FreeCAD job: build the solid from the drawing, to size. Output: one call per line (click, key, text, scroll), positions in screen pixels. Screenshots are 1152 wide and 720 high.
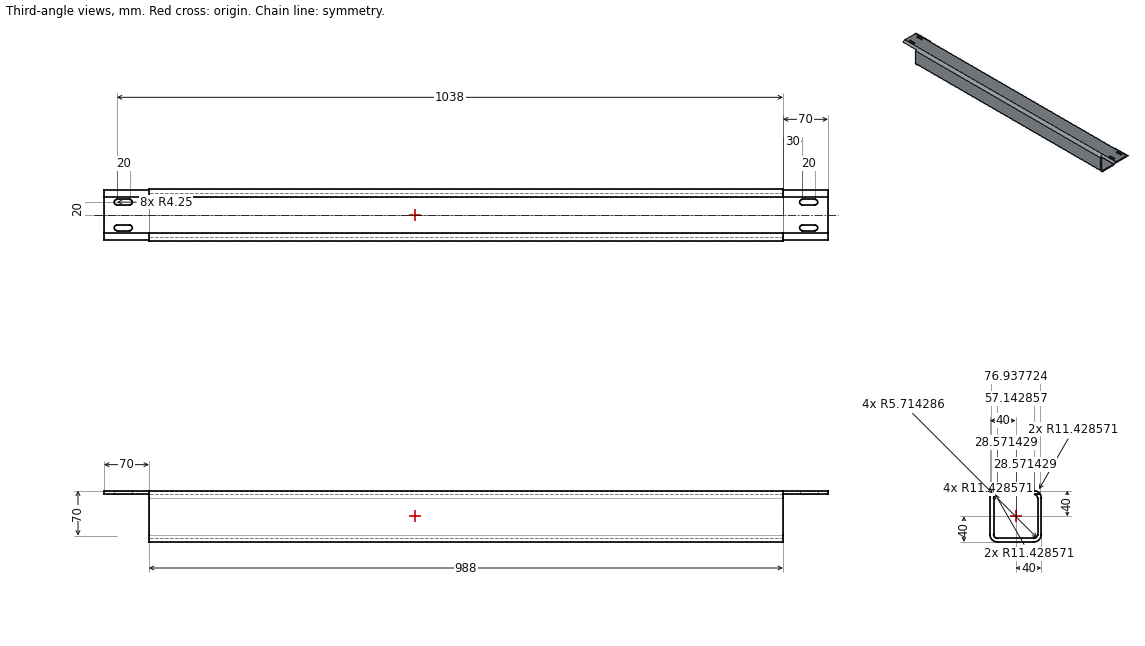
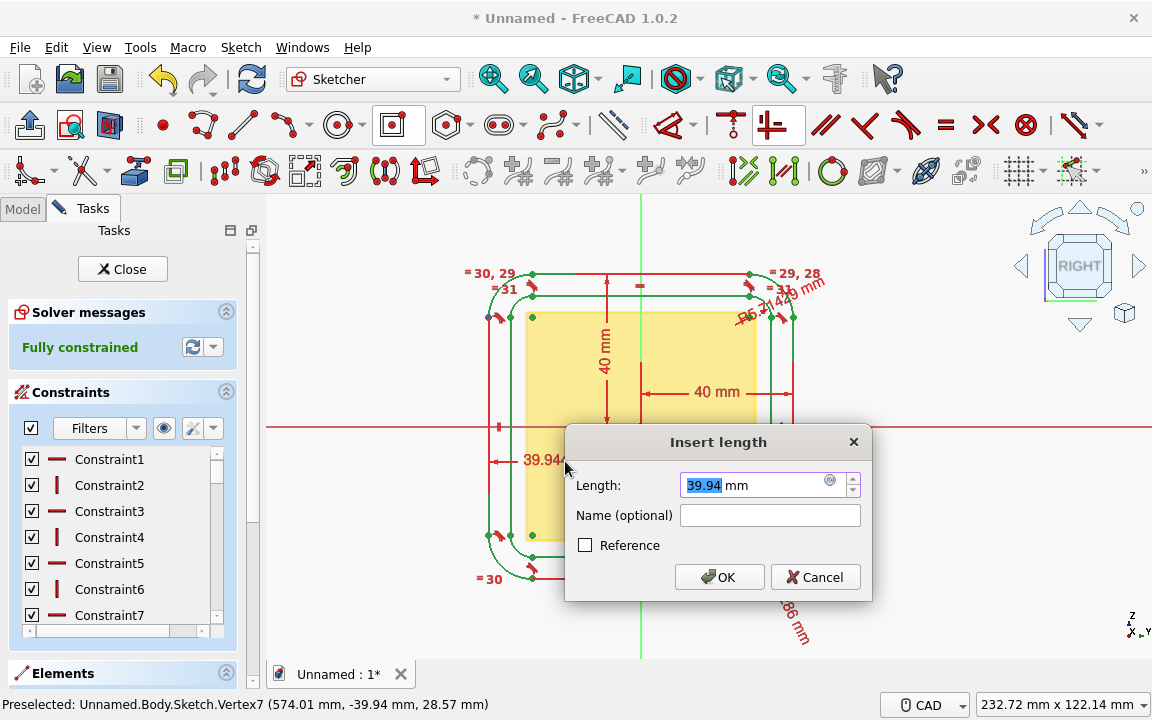
text(40)
key(Return)
key(Escape)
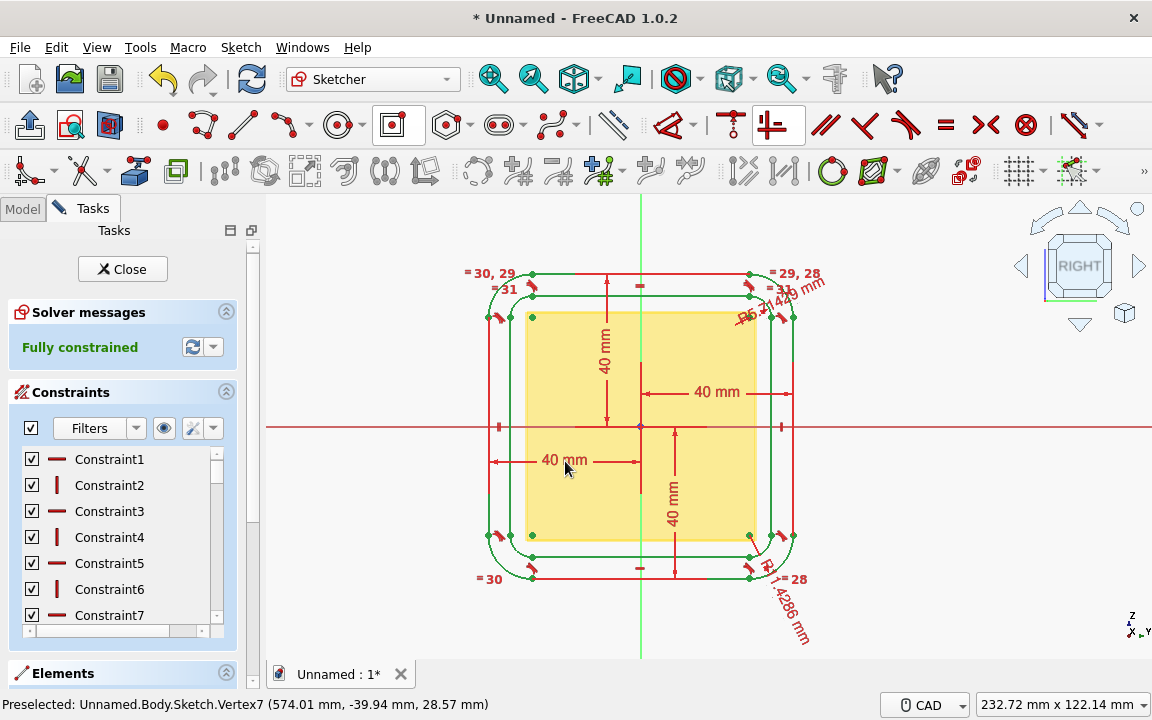
click(123, 269)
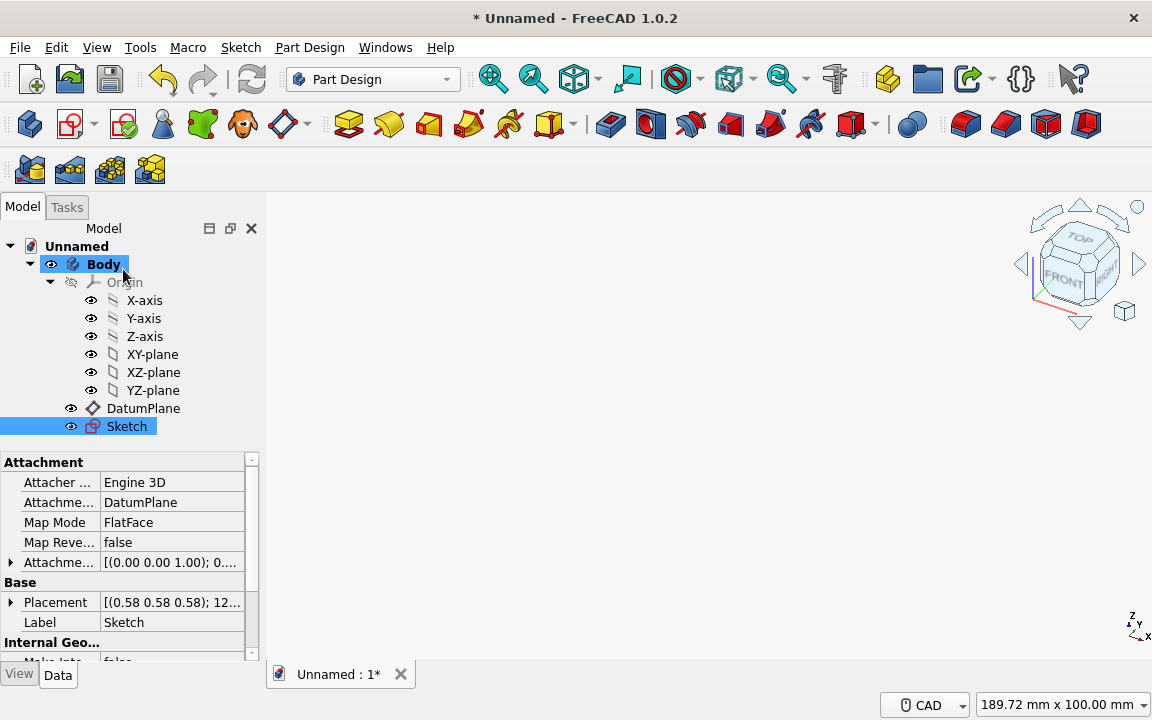
click(350, 124)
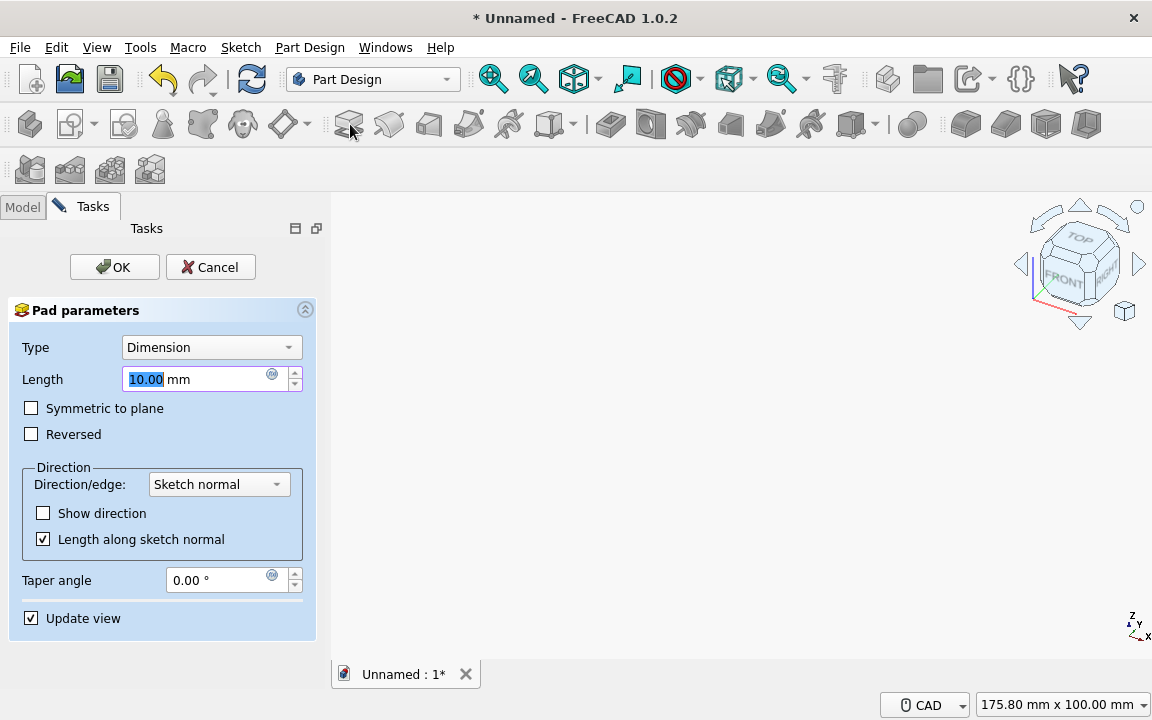
text(988)
key(Tab)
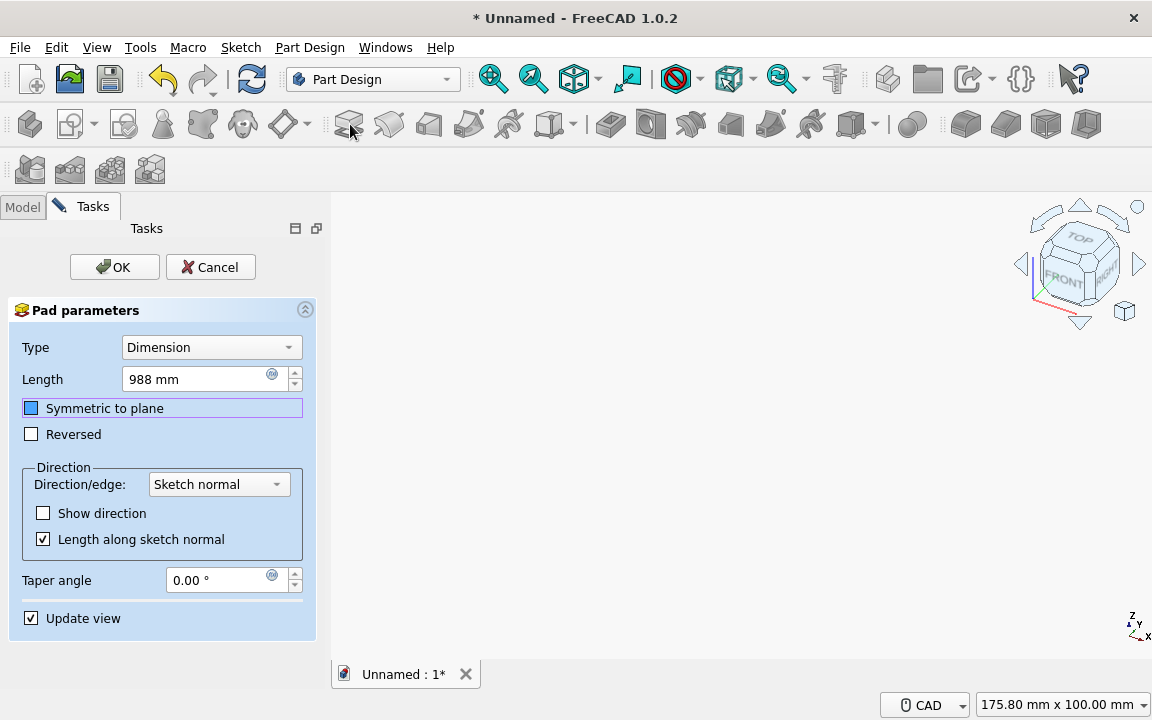
click(30, 434)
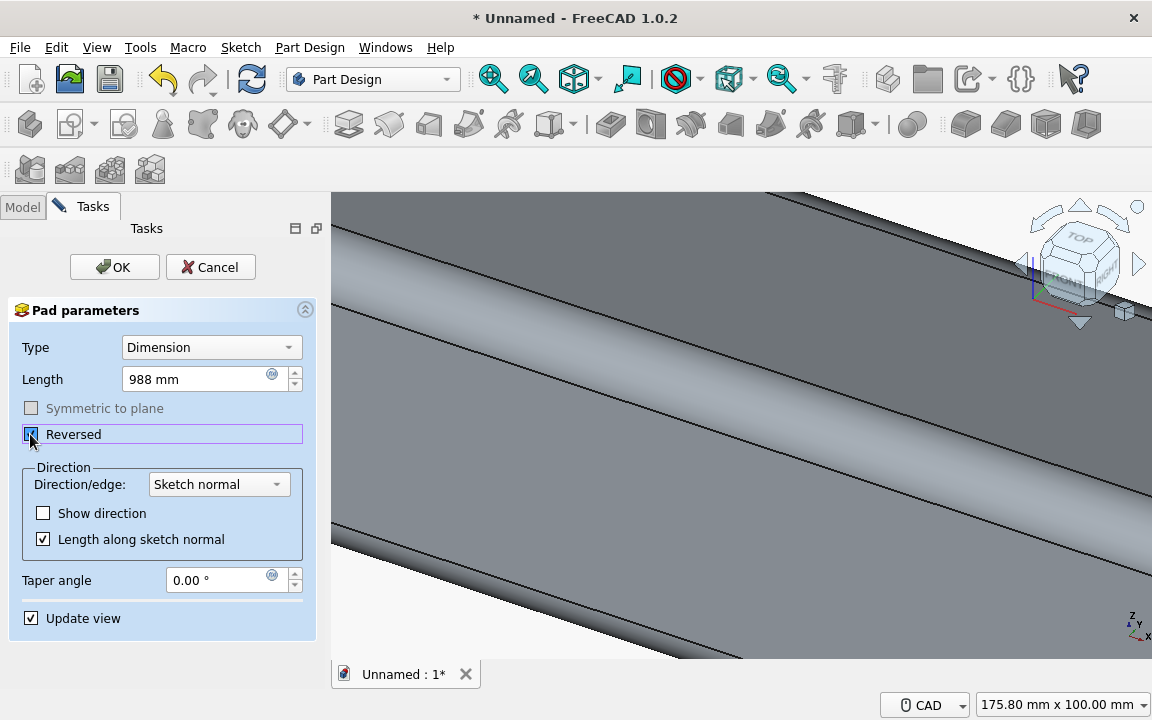
click(115, 267)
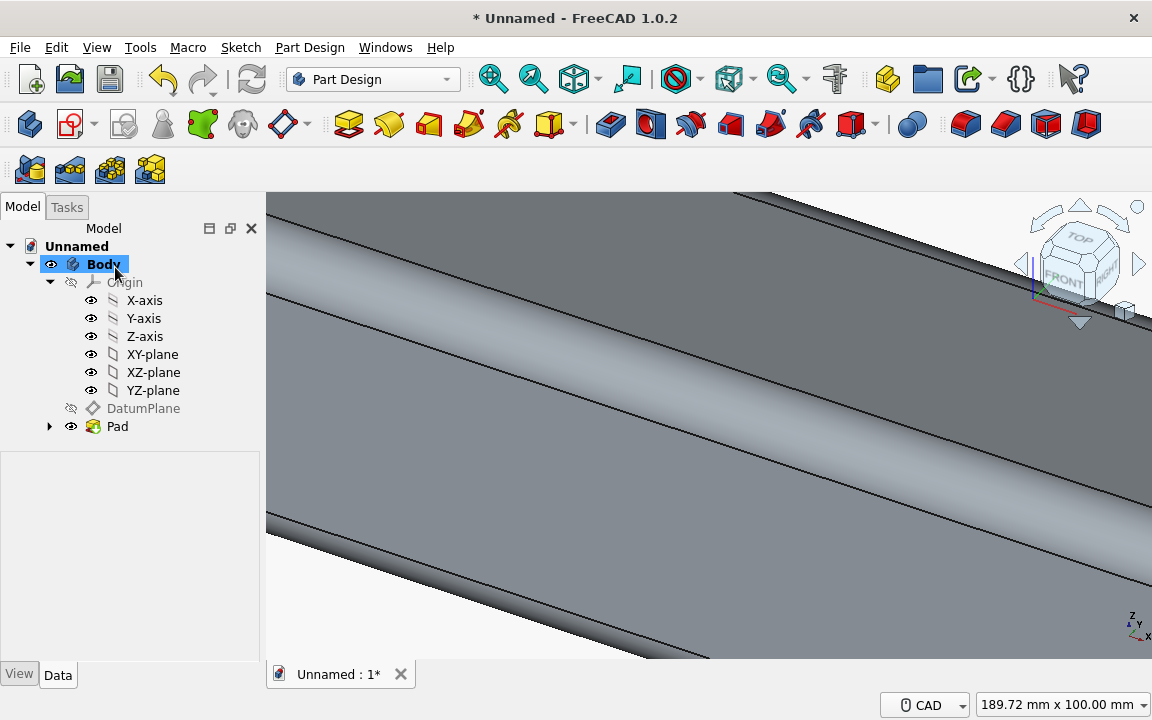
key(v)
key(f)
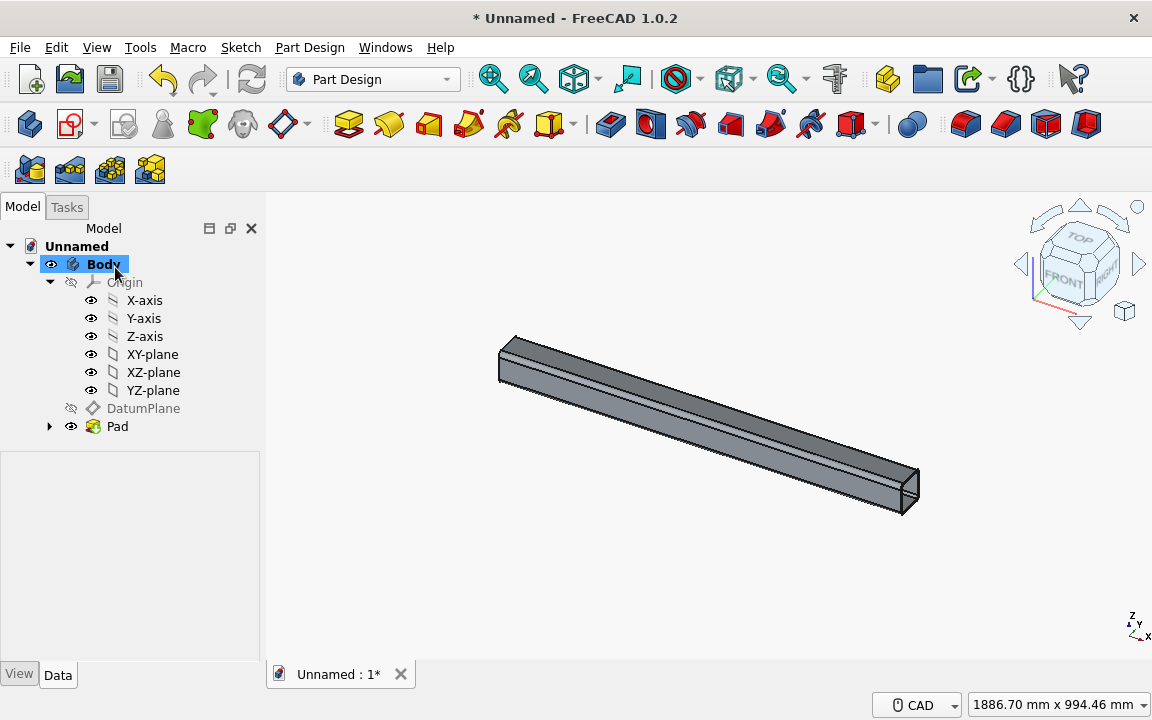
click(136, 390)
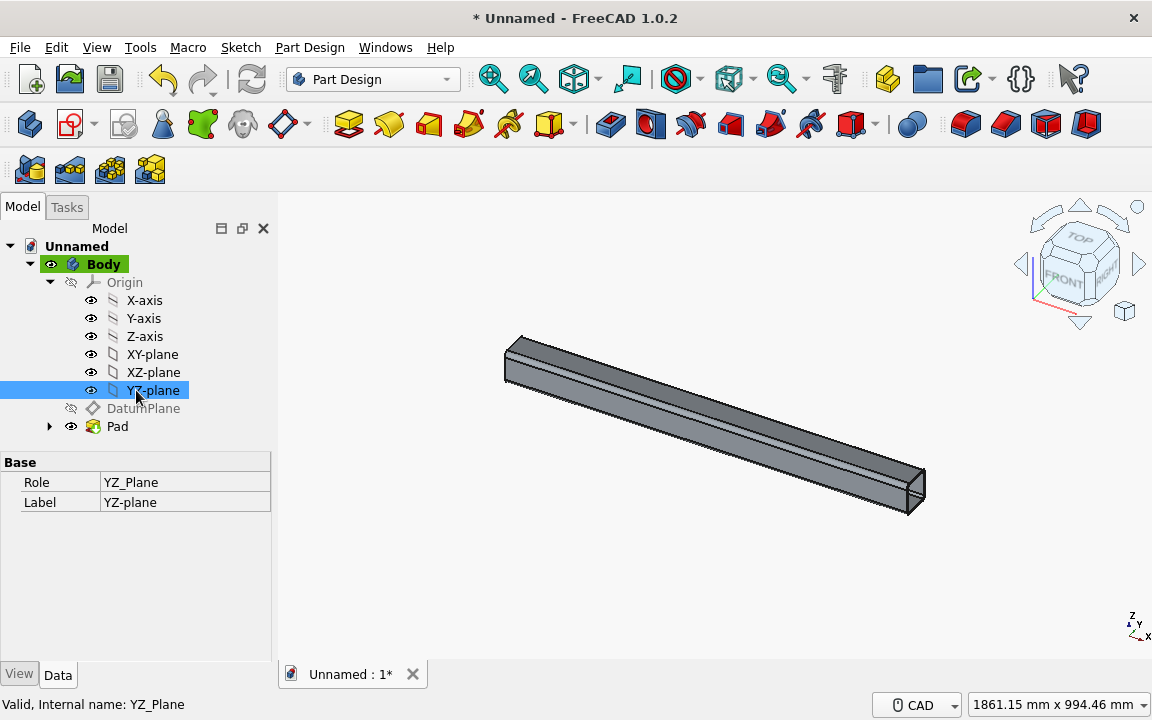
click(284, 124)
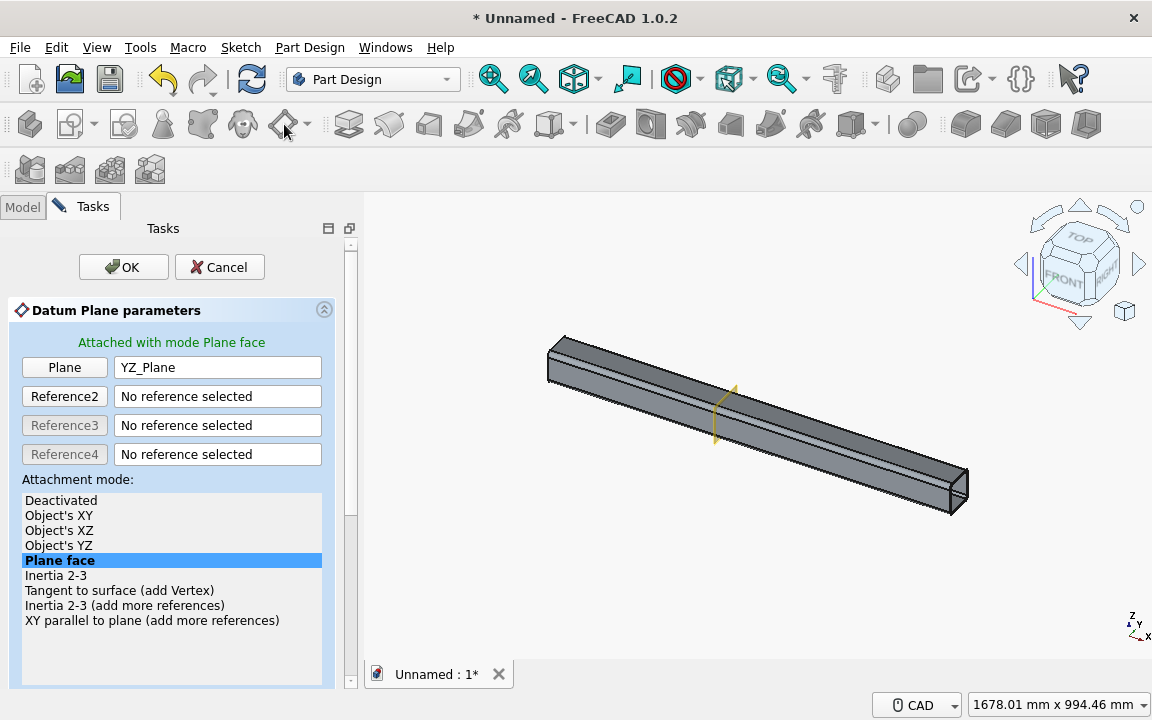
scroll(351, 463, down, 3)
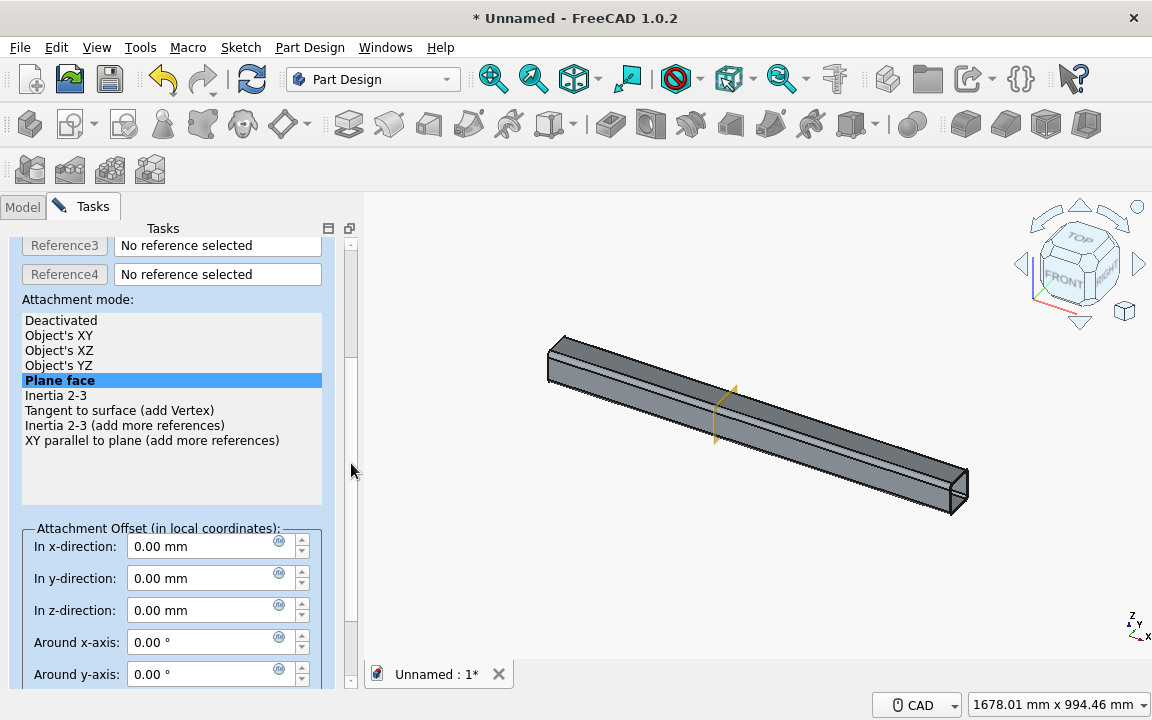
triple_click(210, 610)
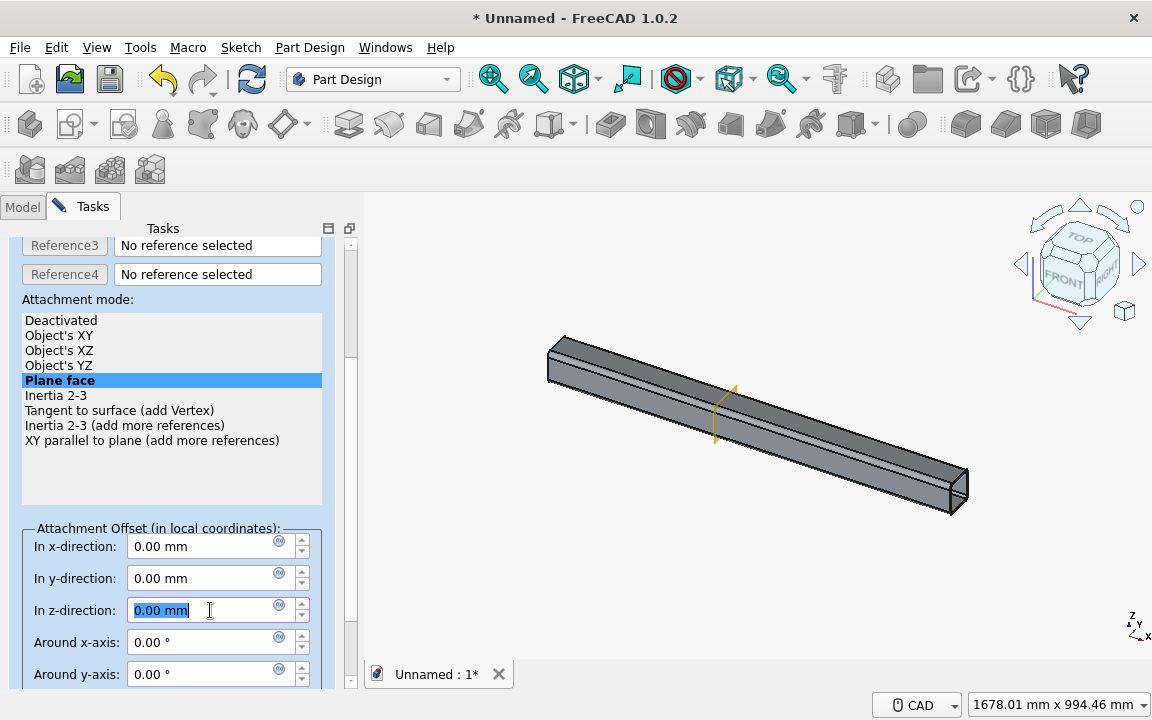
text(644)
key(Tab)